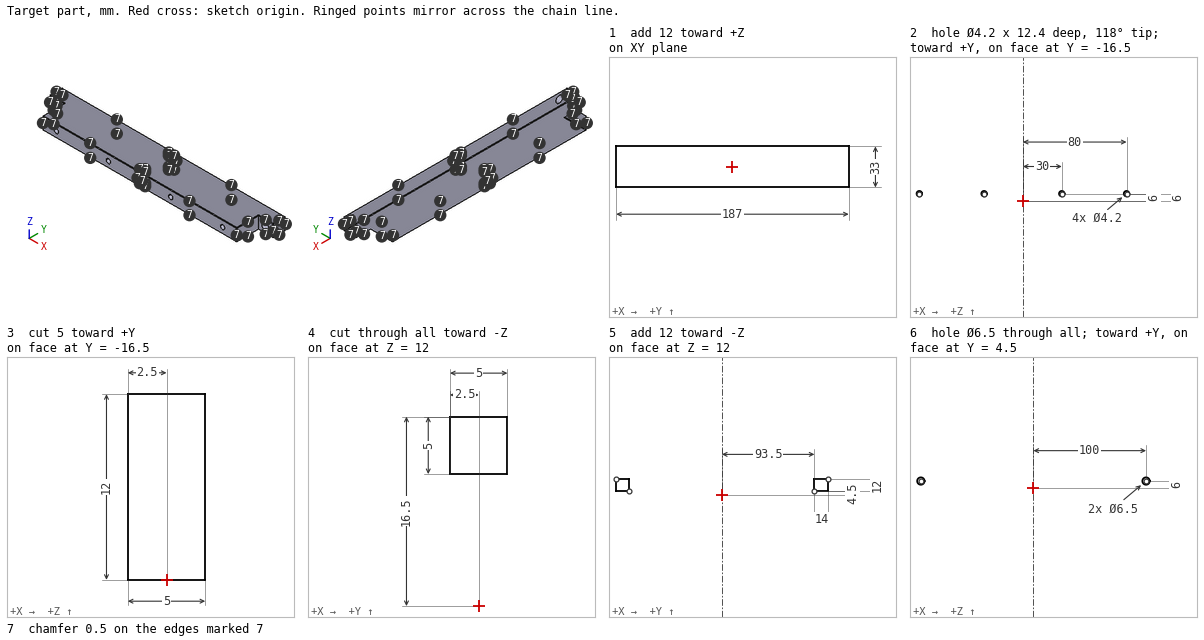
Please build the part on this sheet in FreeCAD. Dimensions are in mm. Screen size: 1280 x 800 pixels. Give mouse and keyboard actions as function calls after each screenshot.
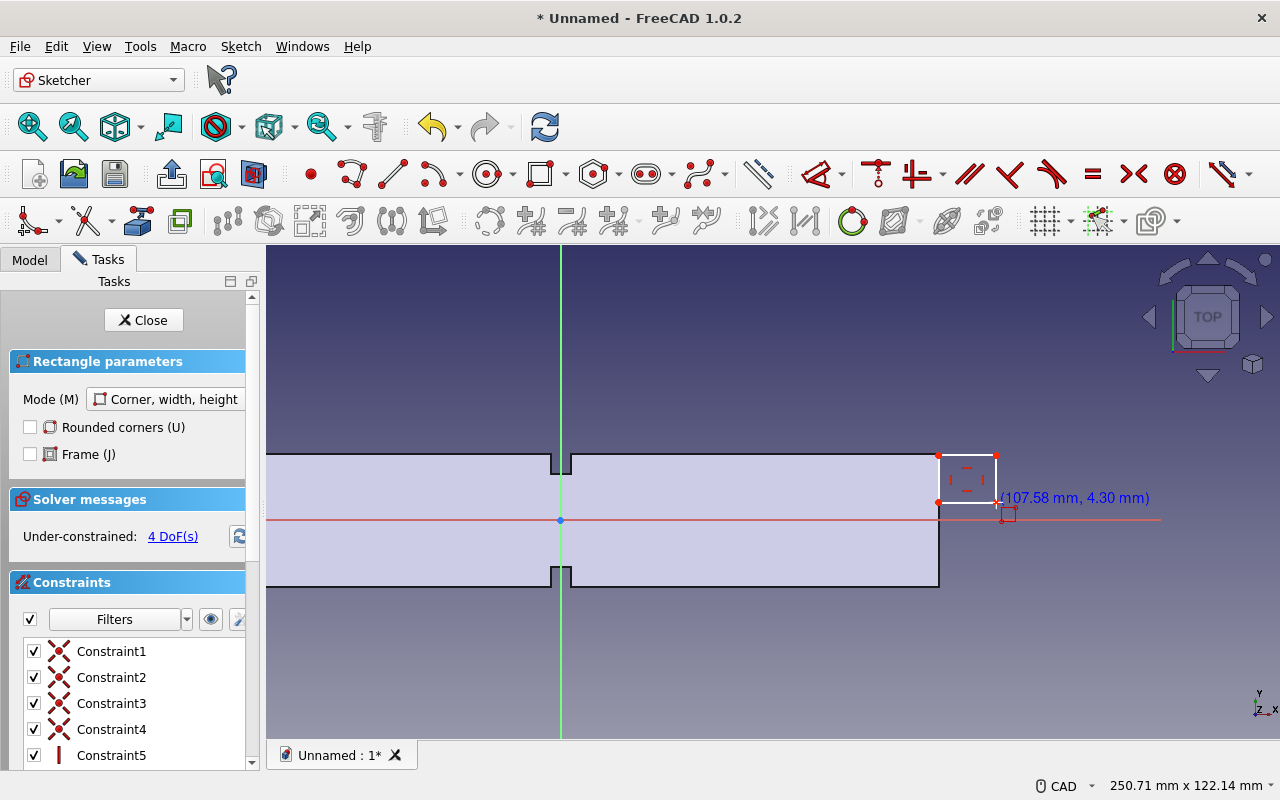
scroll(996, 502, down, 2)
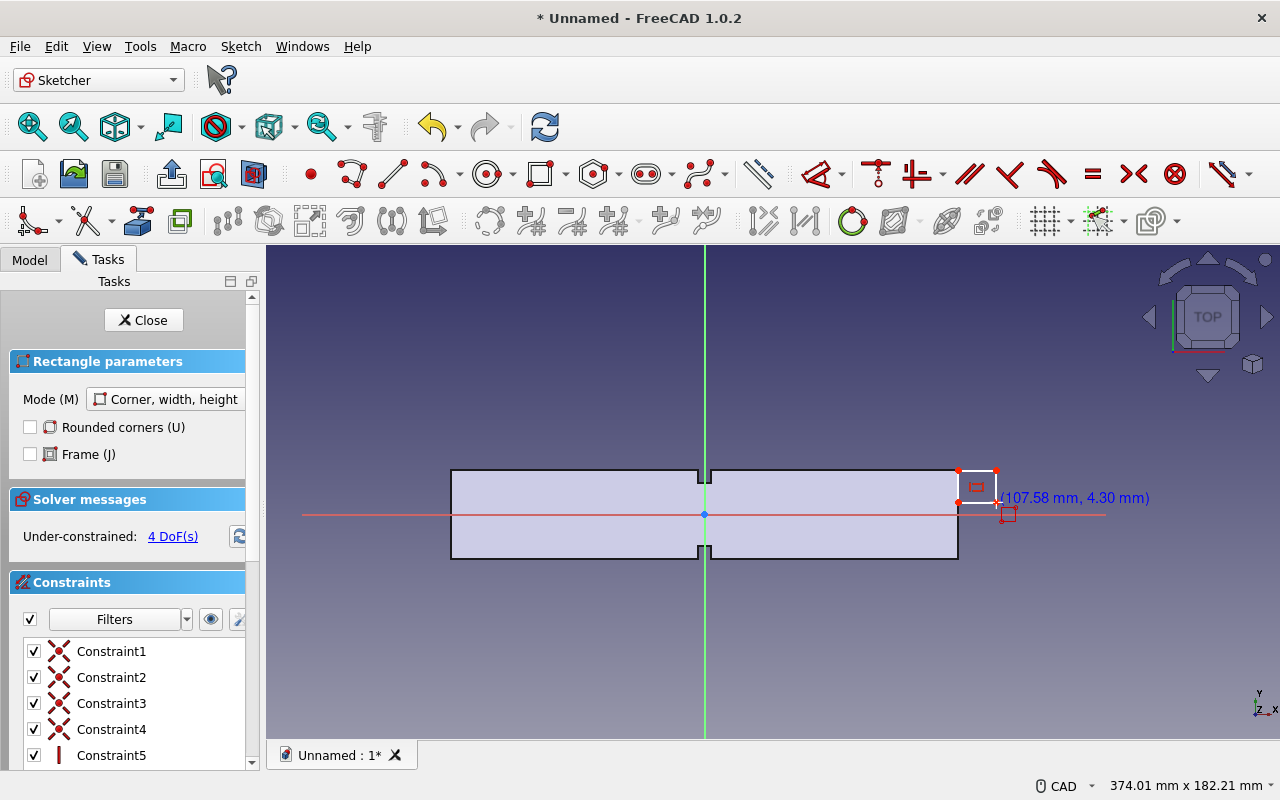
click(413, 470)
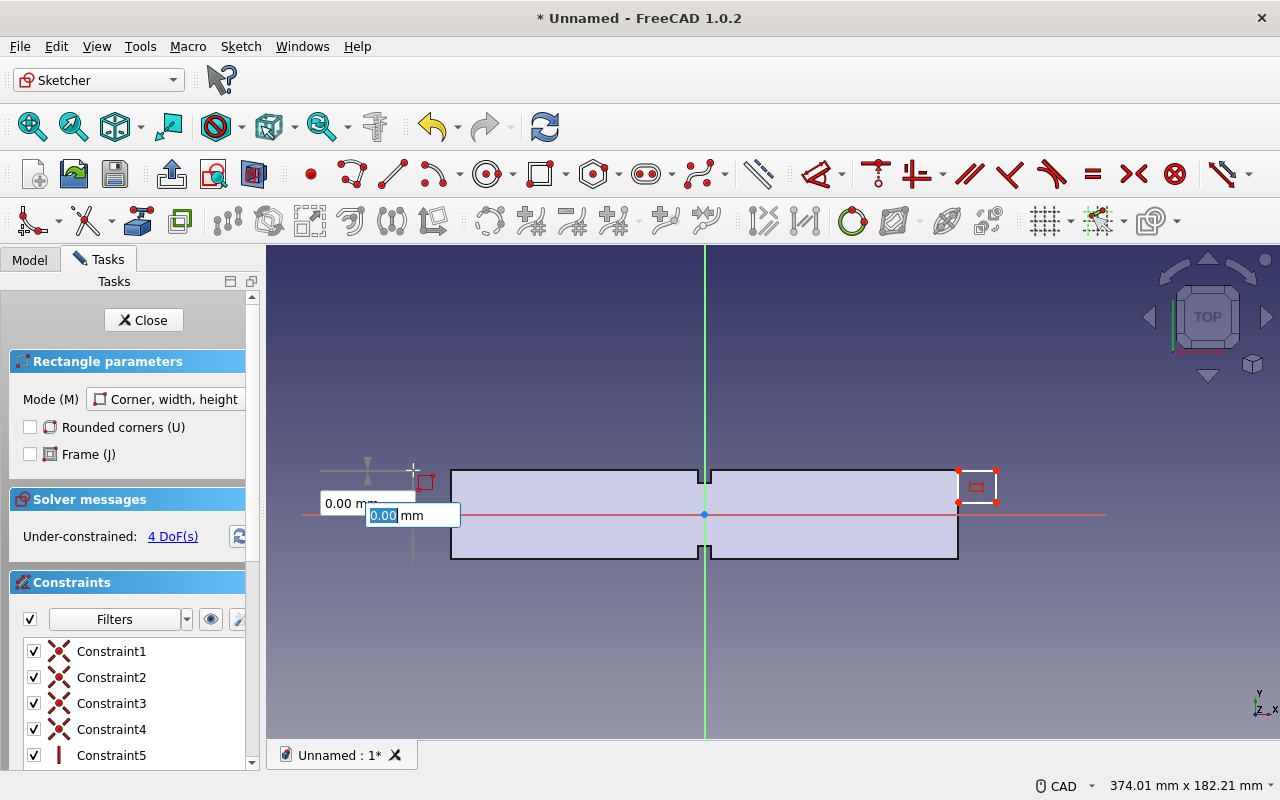
scroll(451, 502, up, 2)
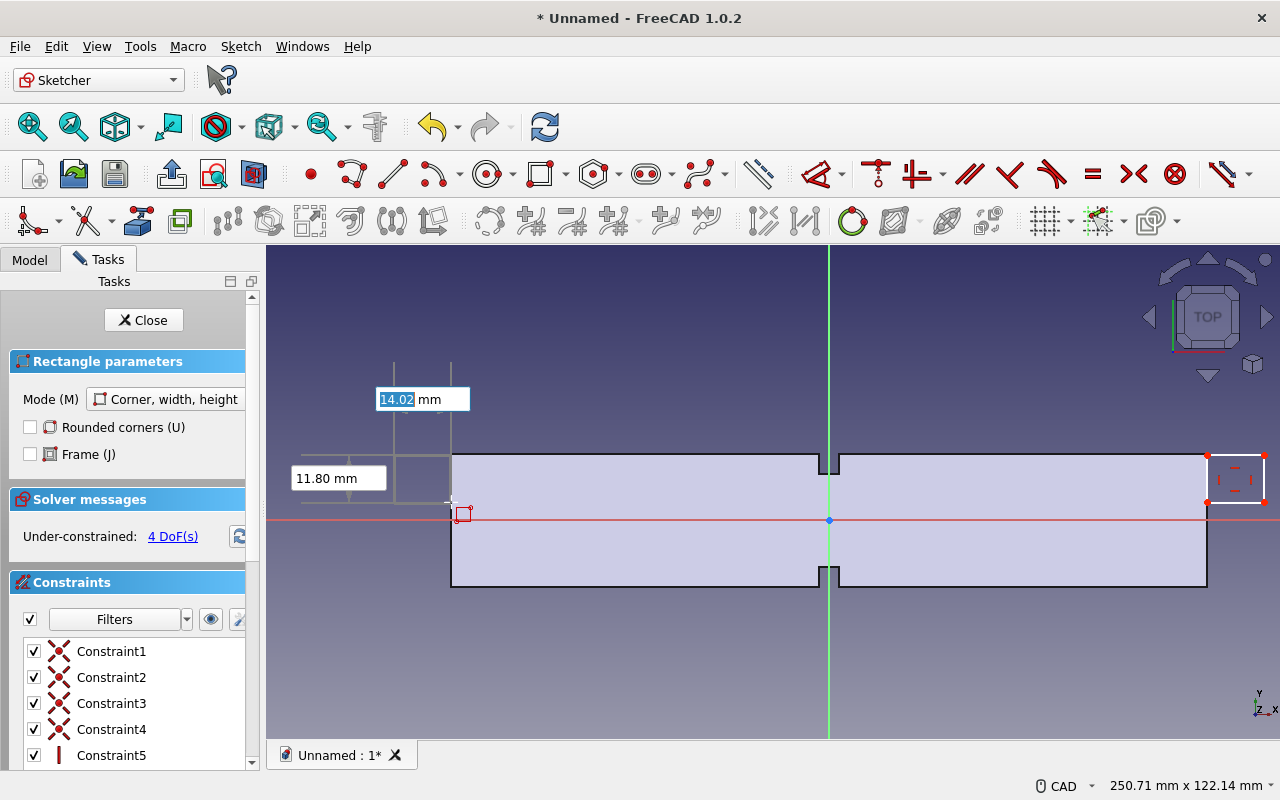
click(451, 502)
key(Escape)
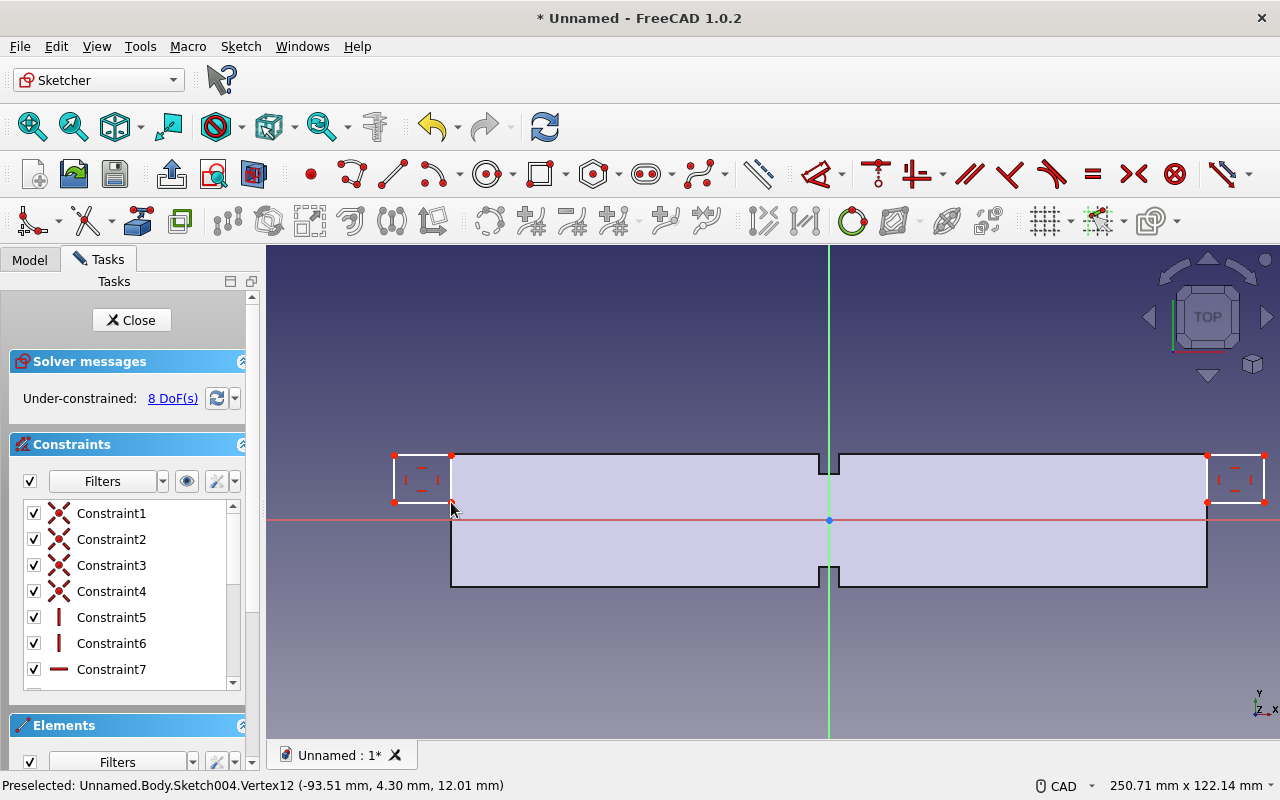
scroll(451, 502, down, 2)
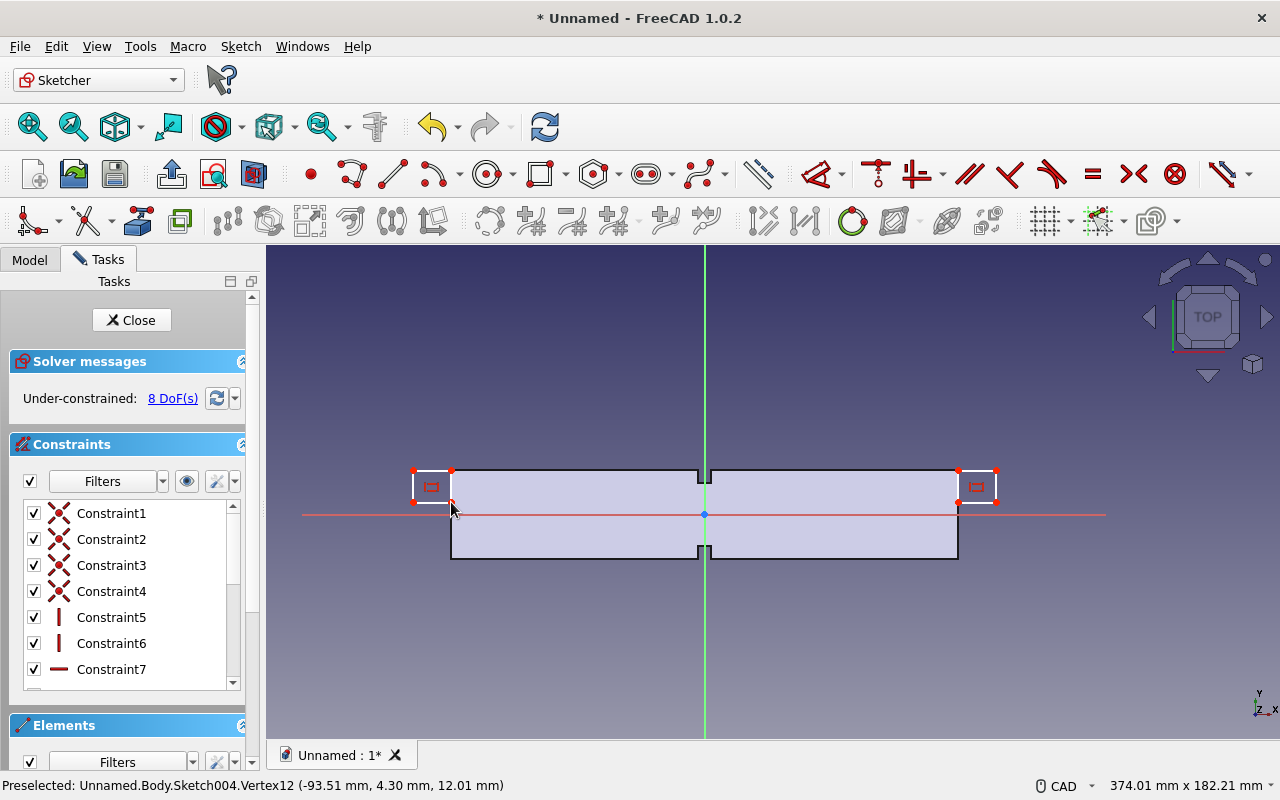
click(996, 471)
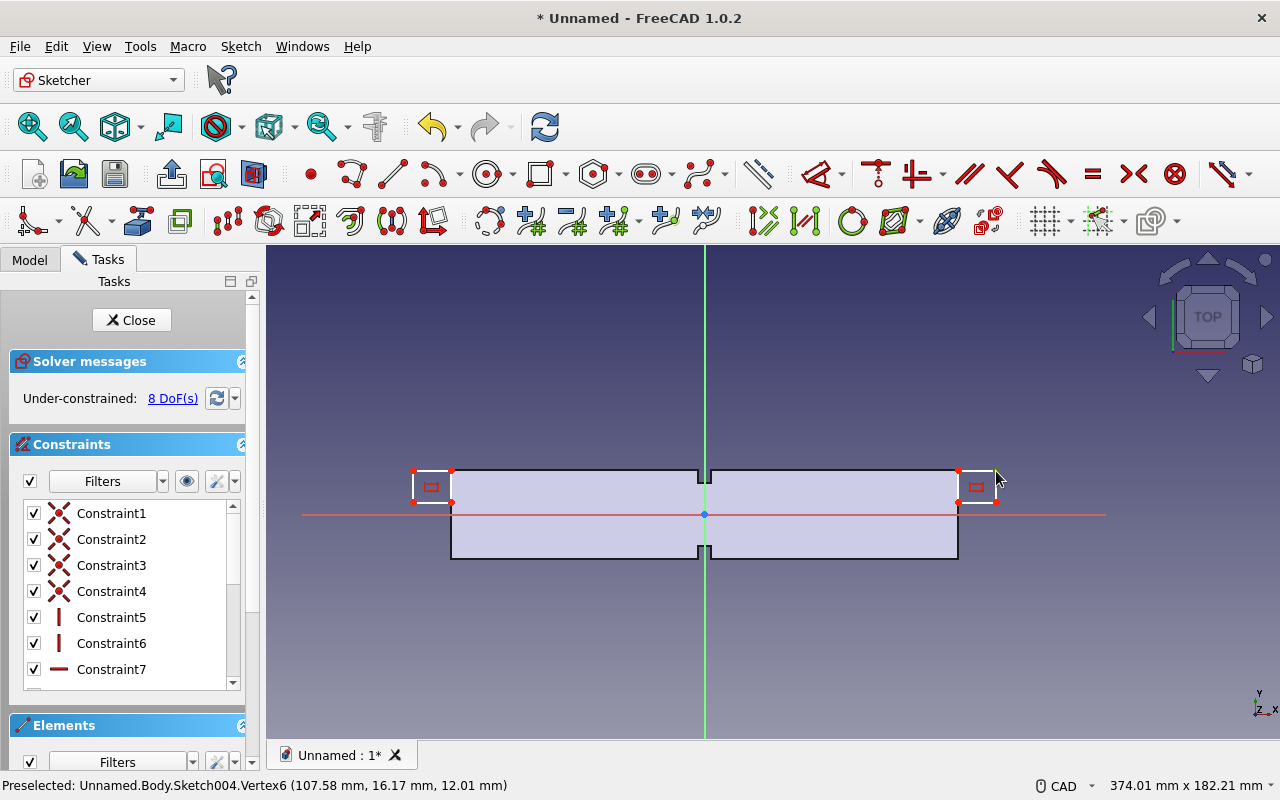
click(413, 471)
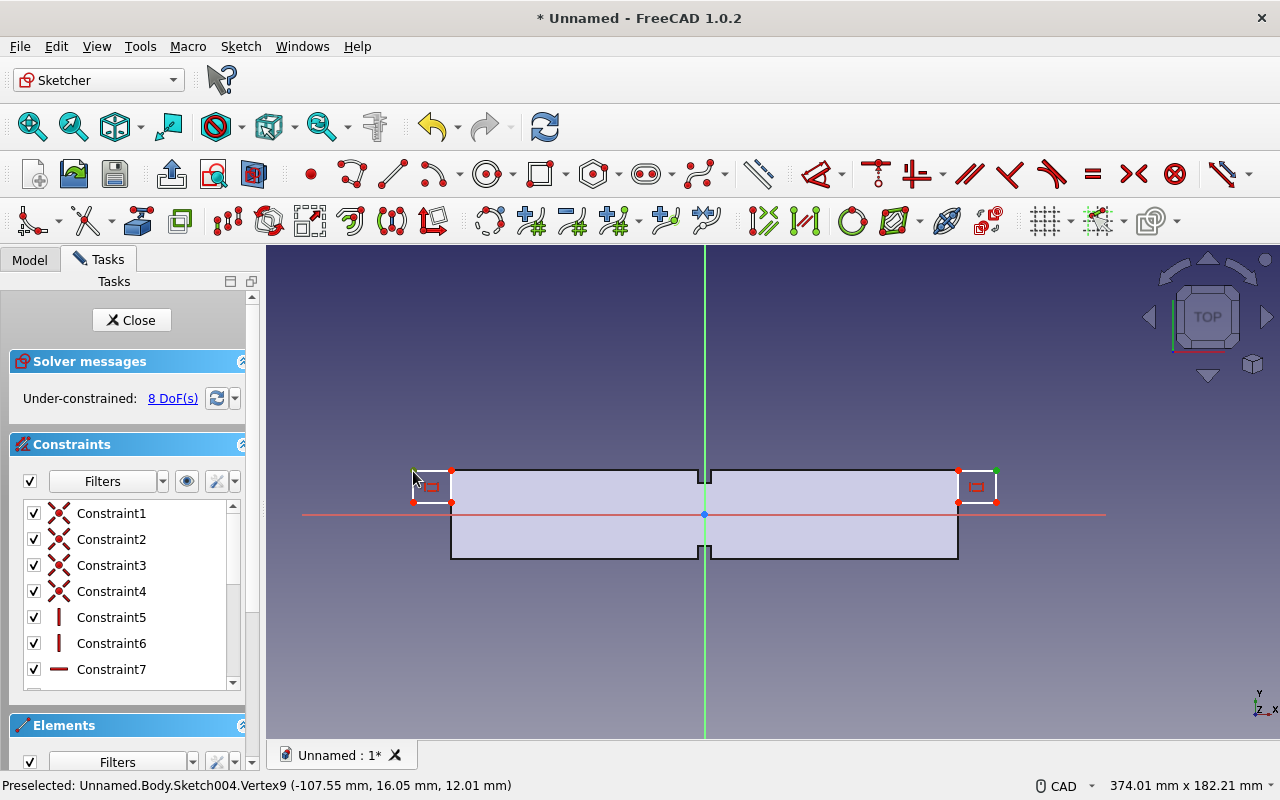
click(705, 680)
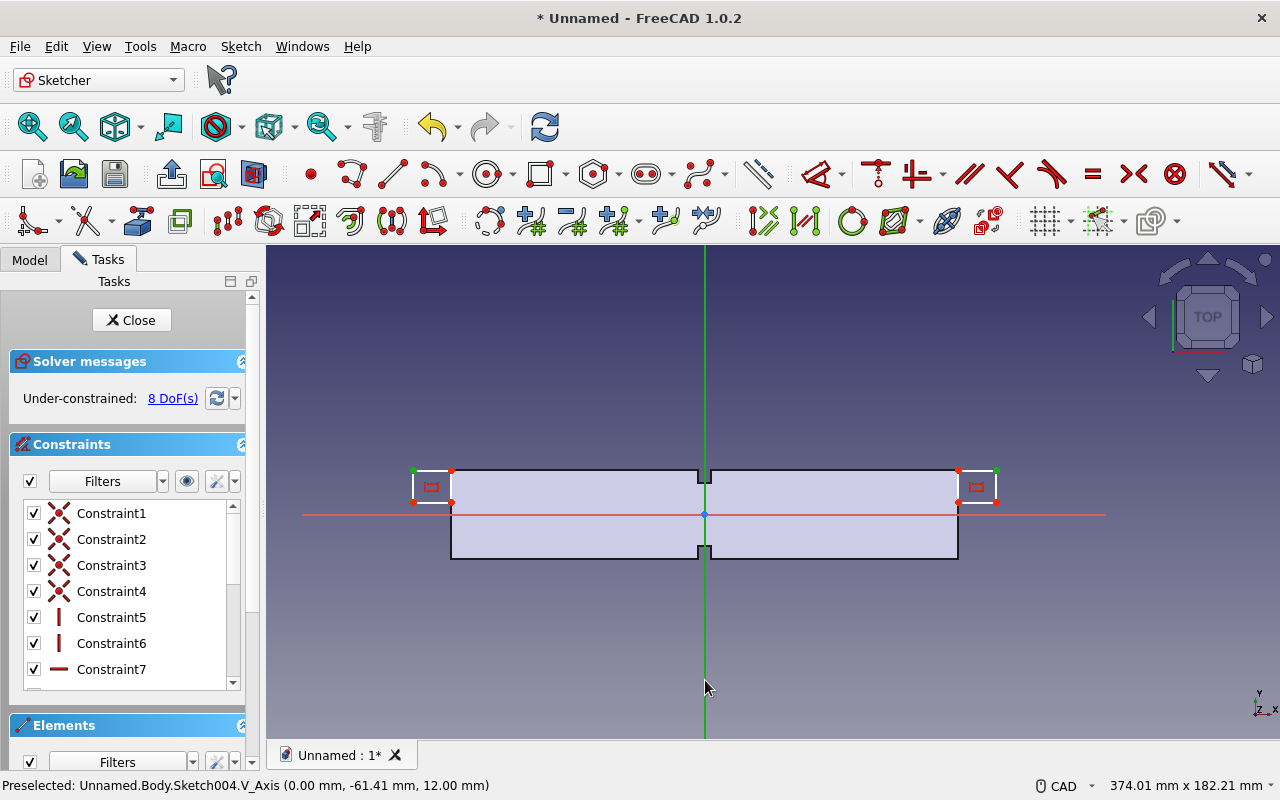
key(s)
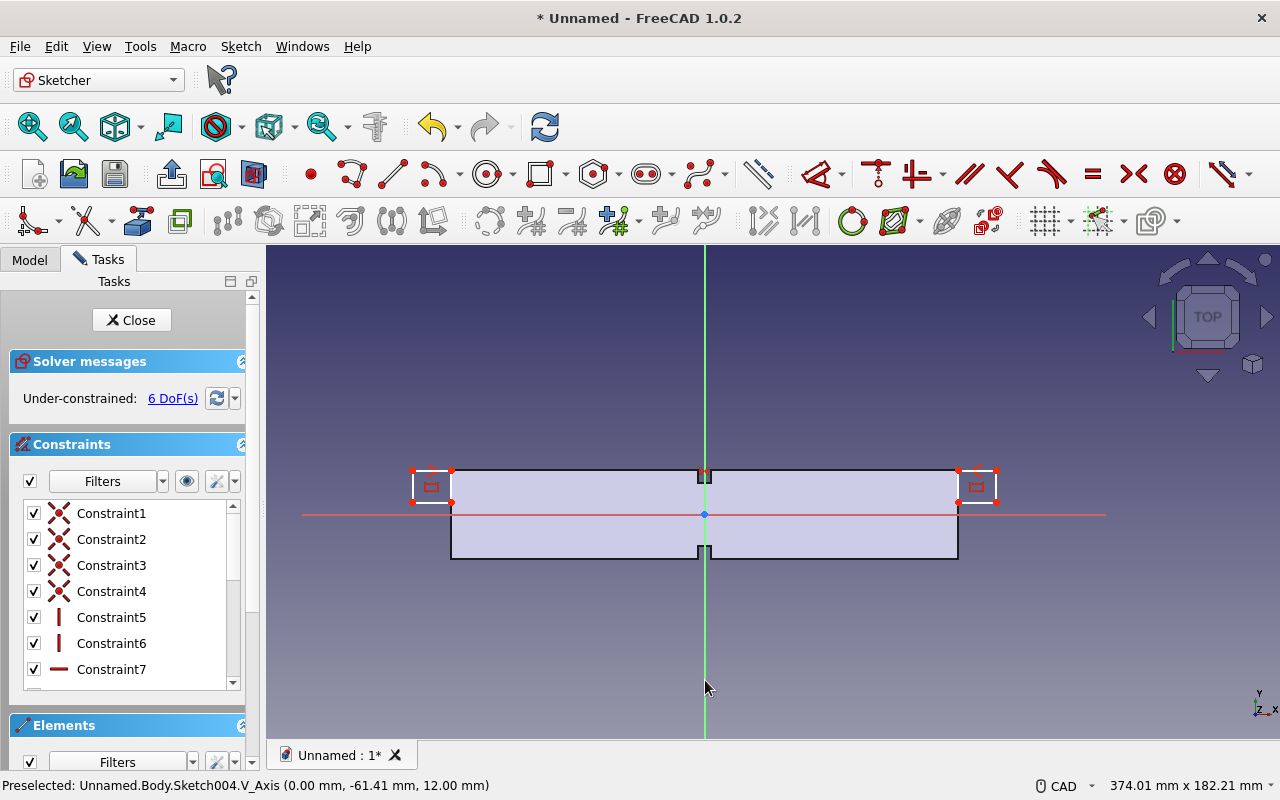
click(958, 503)